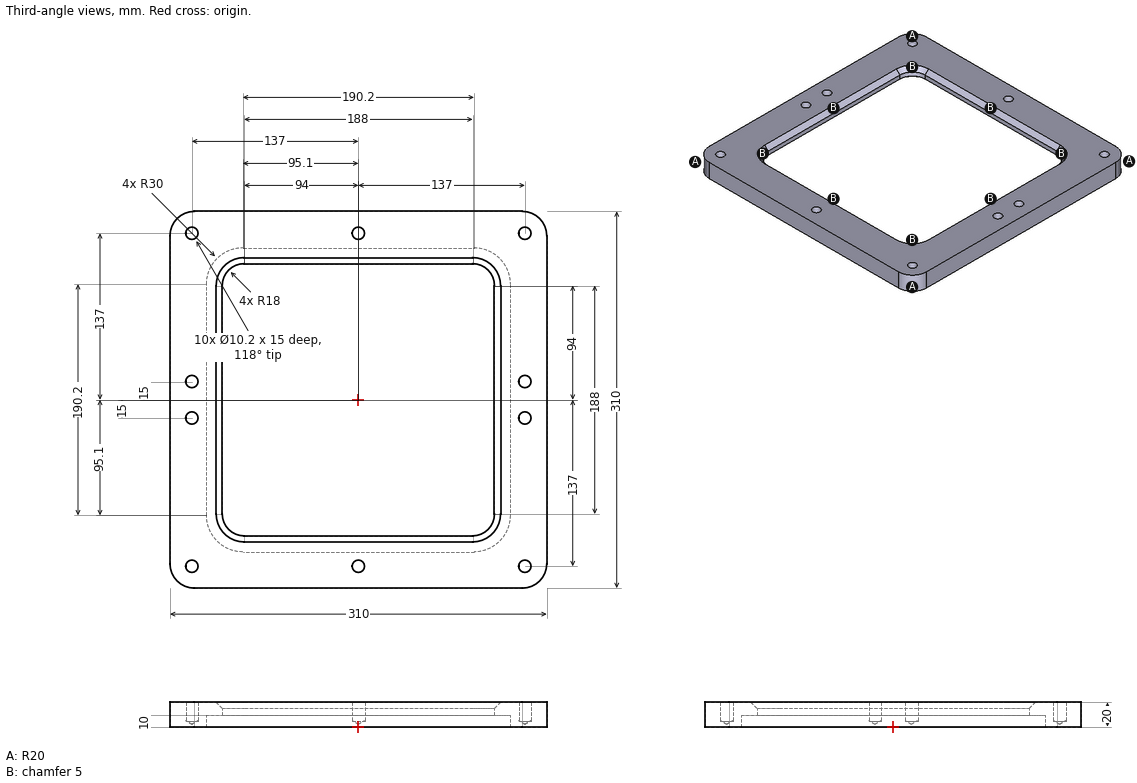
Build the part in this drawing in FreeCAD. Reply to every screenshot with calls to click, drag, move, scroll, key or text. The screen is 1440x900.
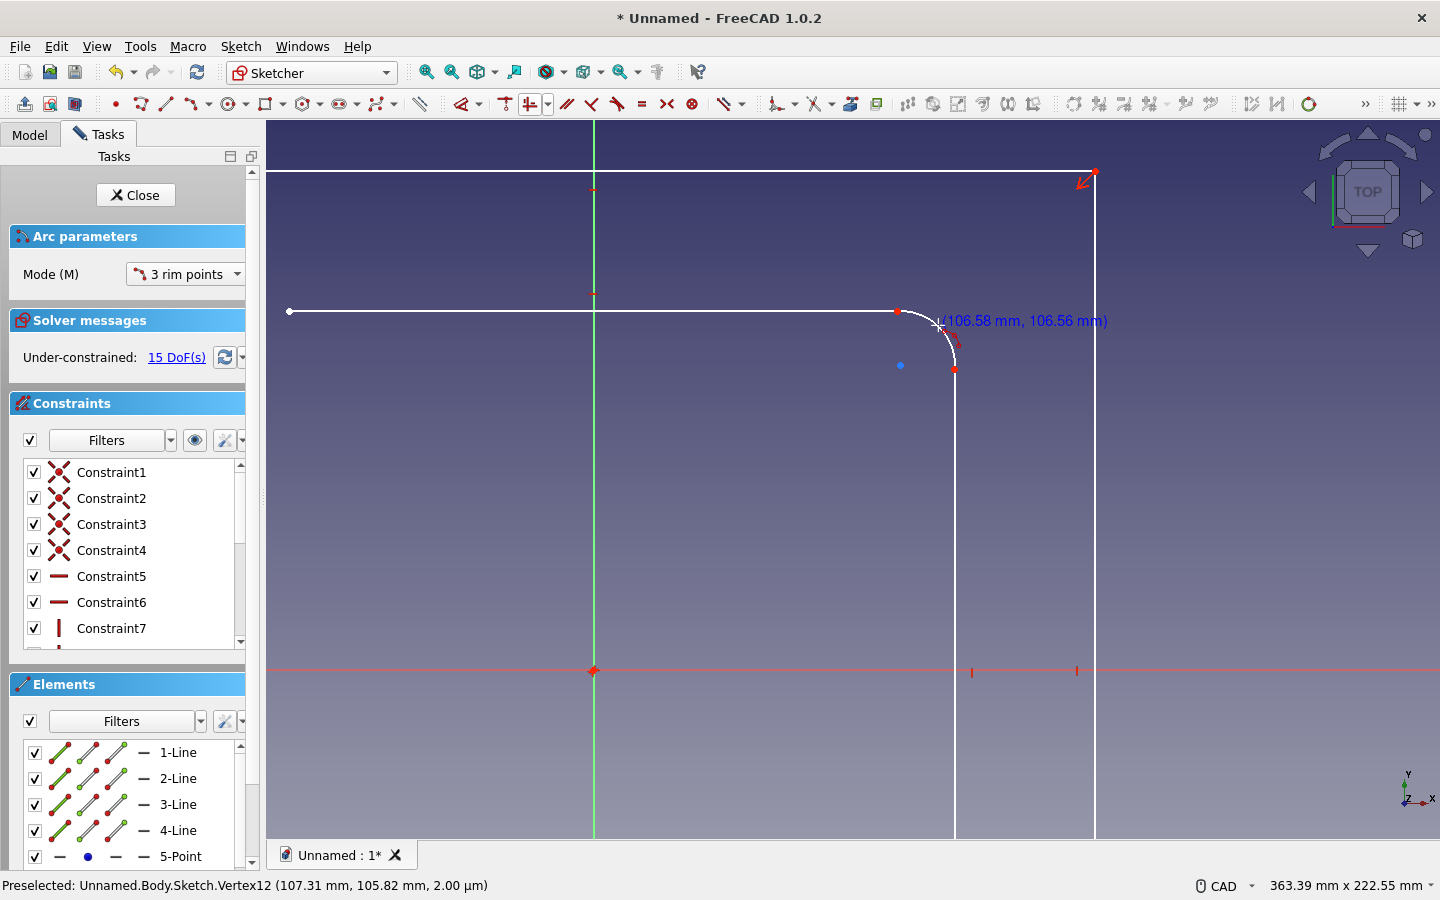
scroll(940, 324, down, 4)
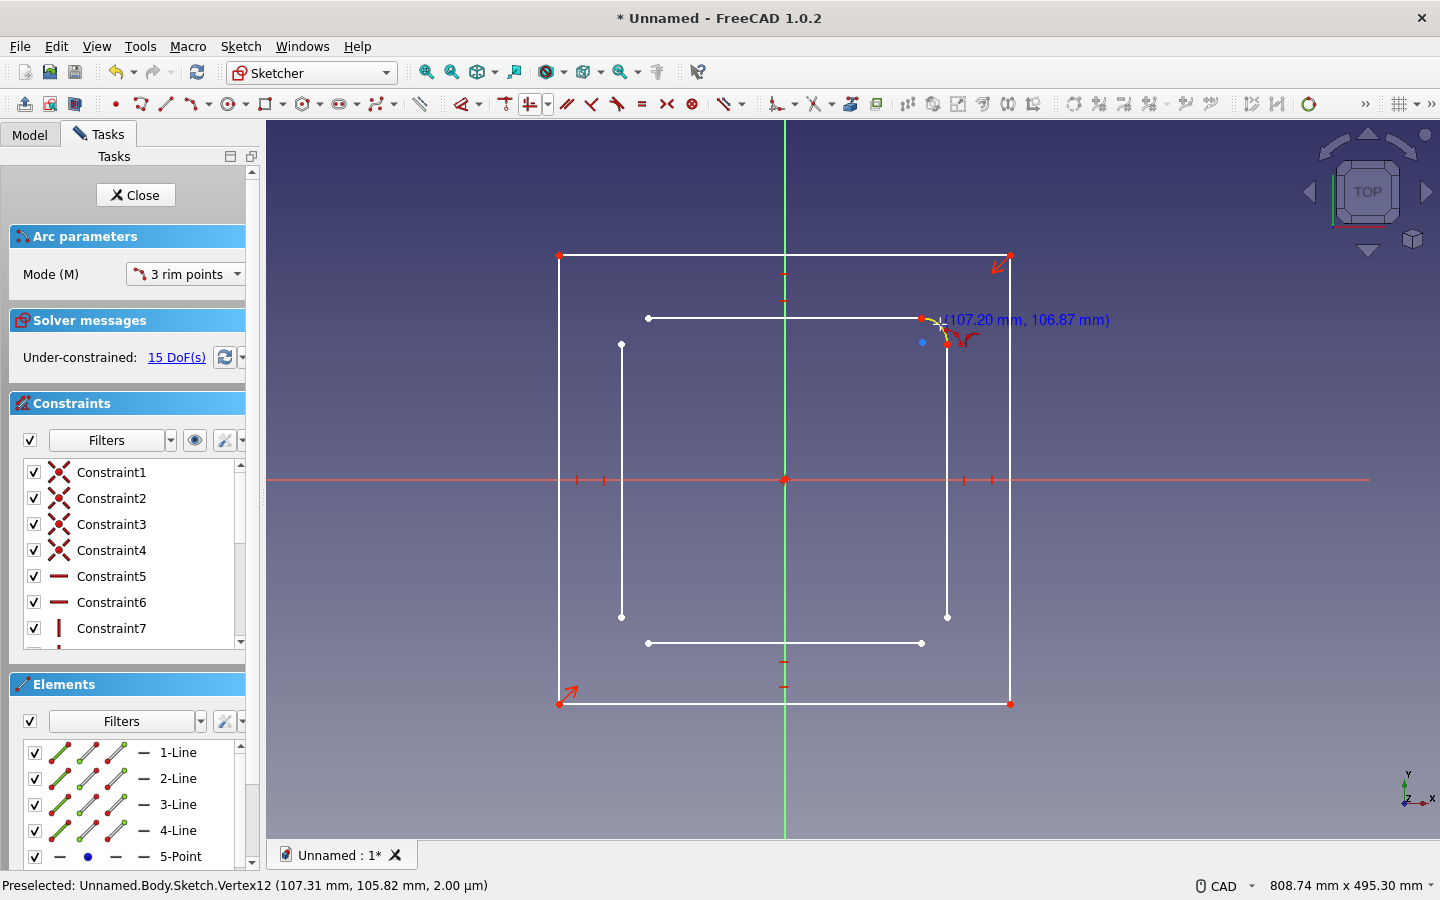
click(947, 617)
click(921, 643)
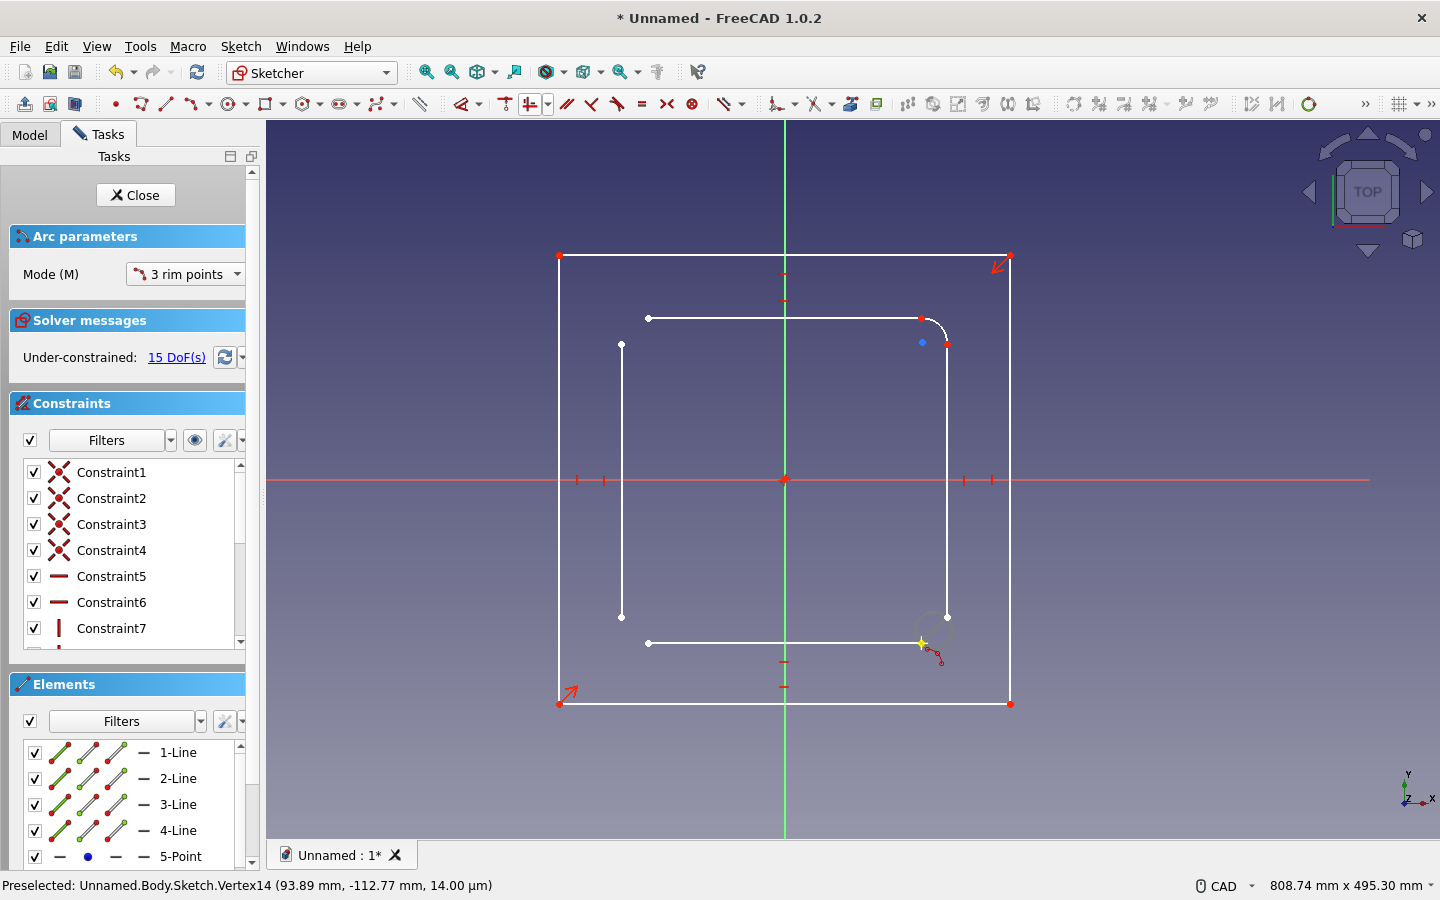
scroll(940, 635, up, 4)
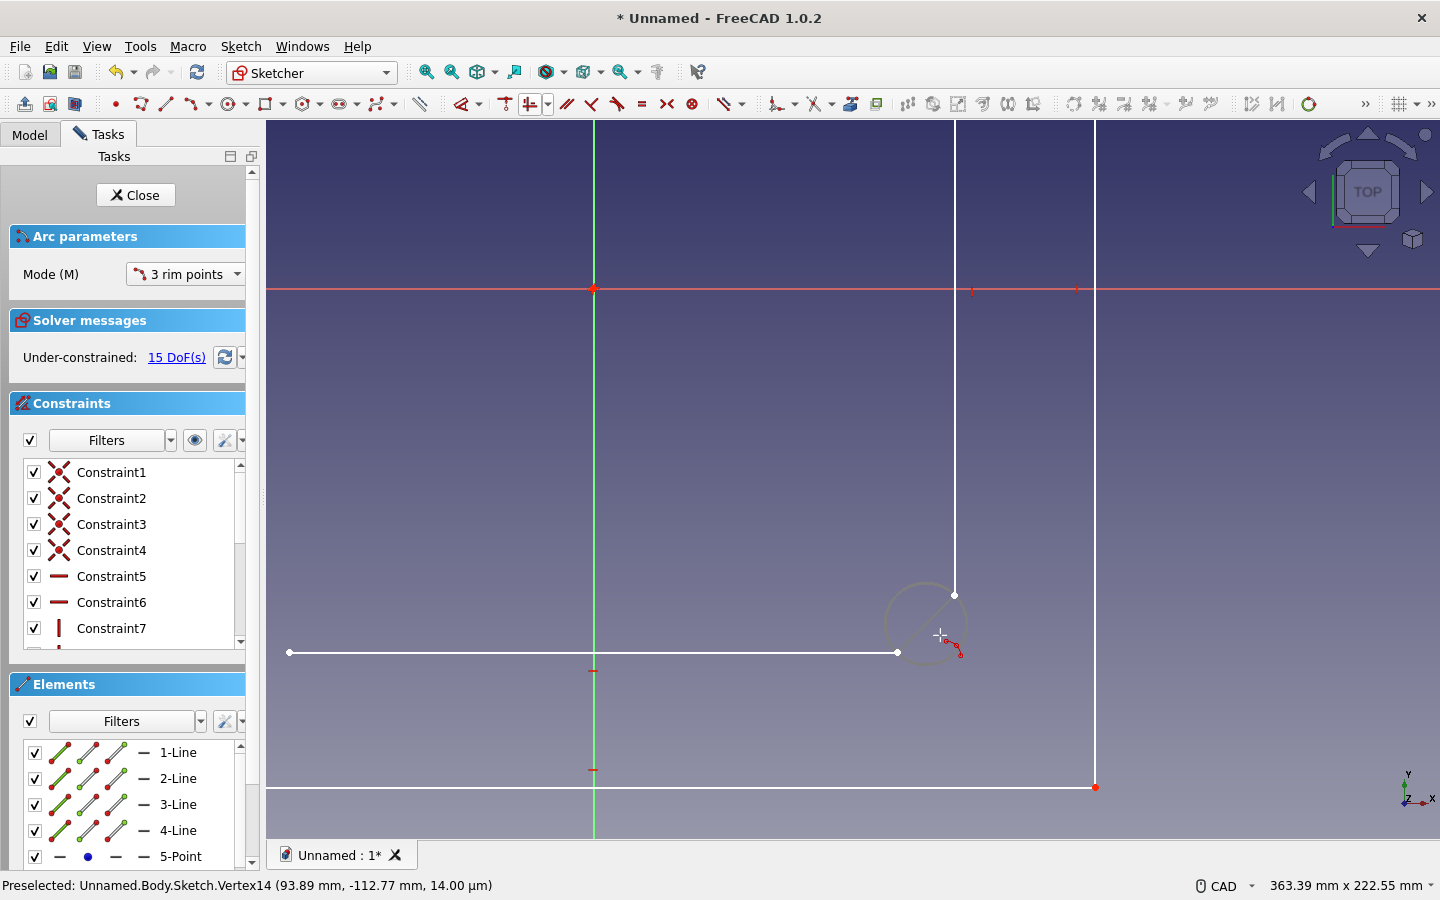
click(938, 633)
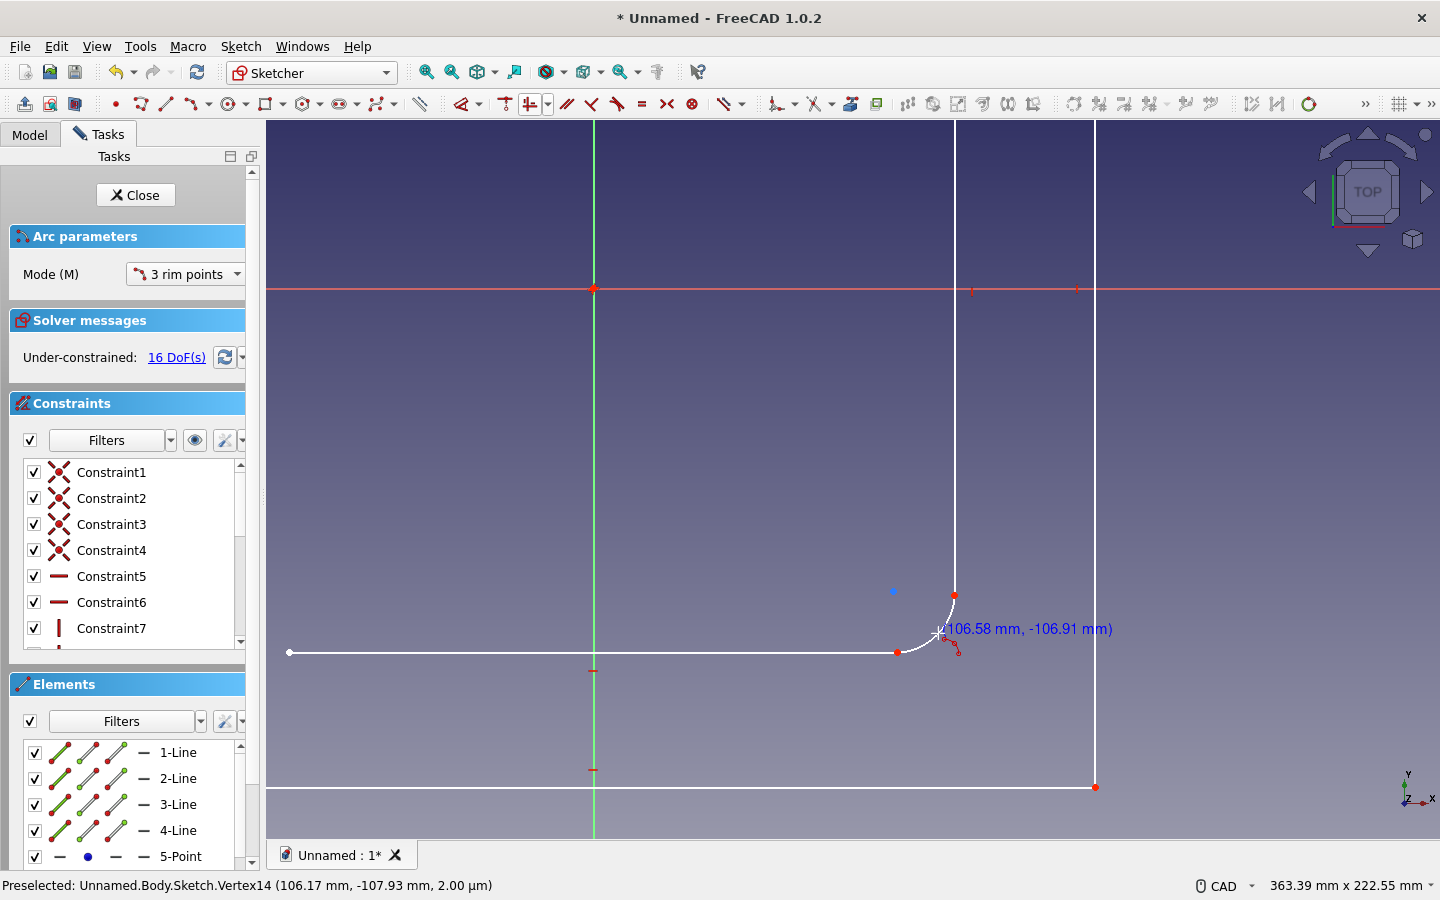
scroll(940, 635, down, 4)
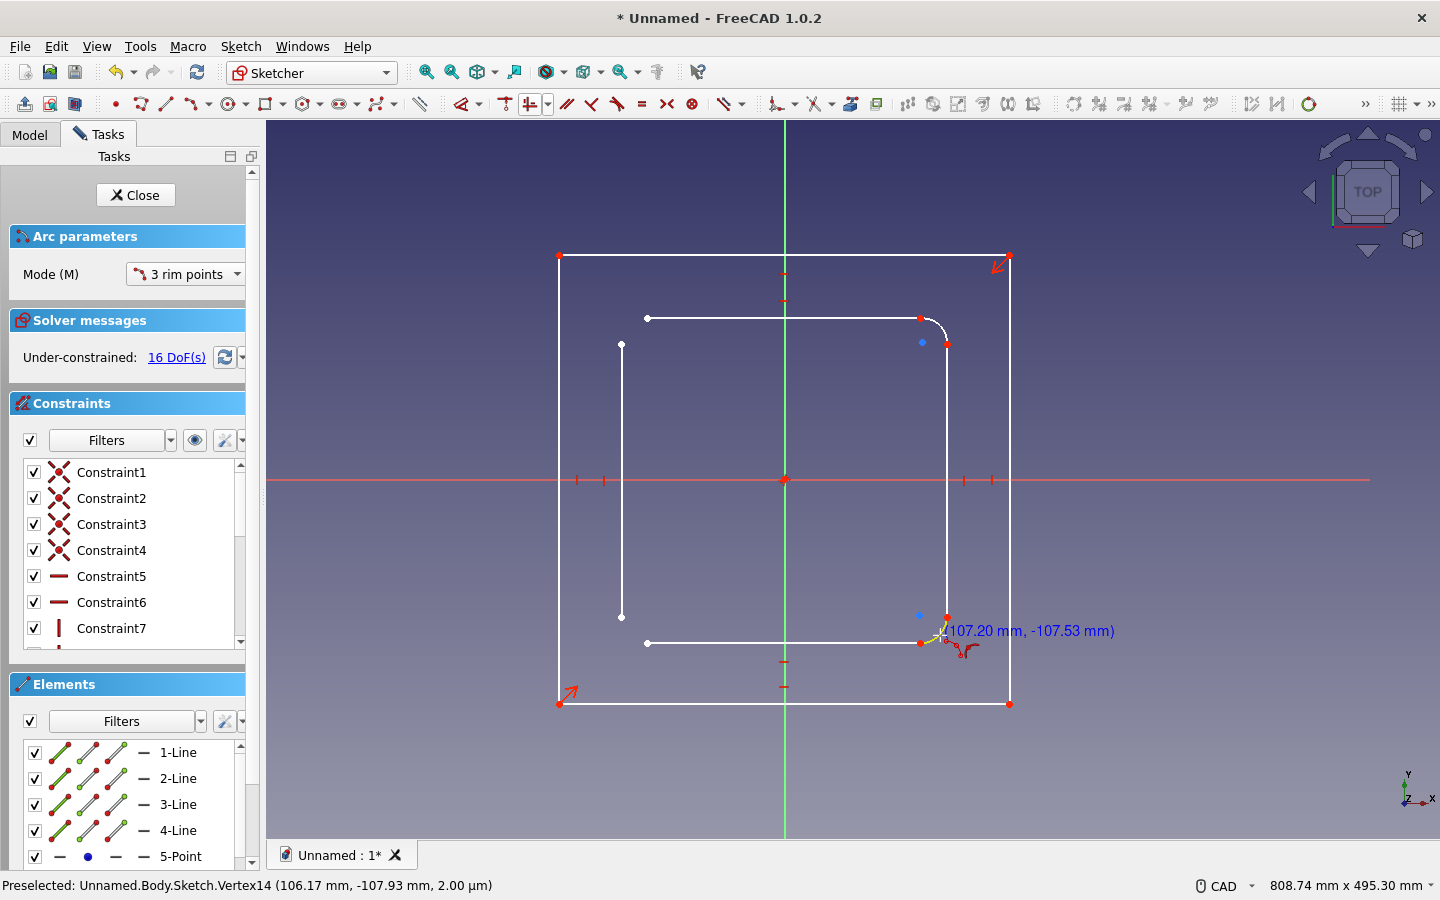
click(648, 643)
click(622, 617)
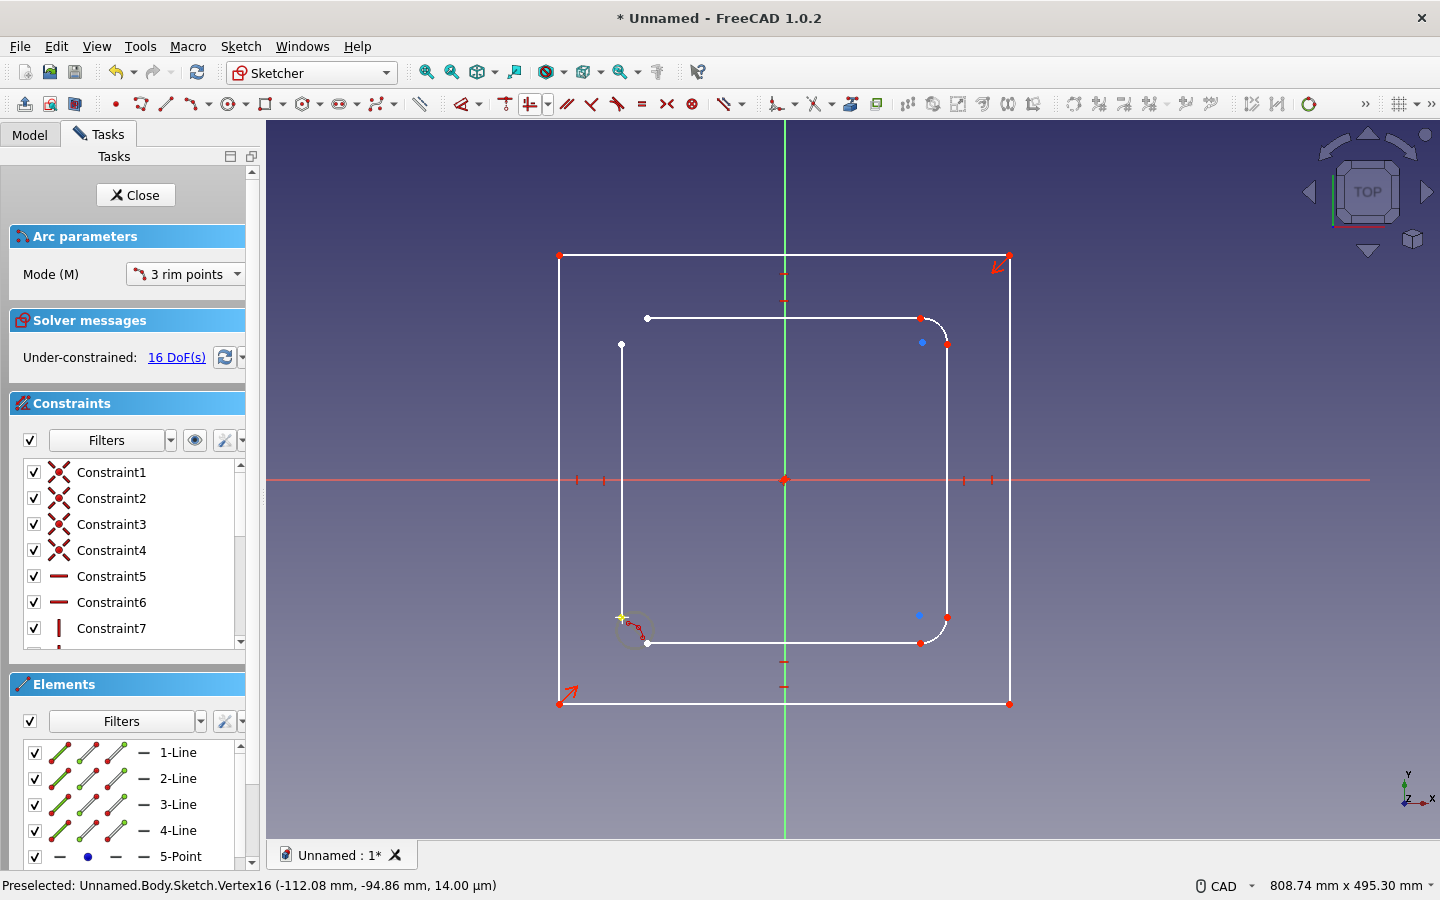
scroll(630, 635, up, 4)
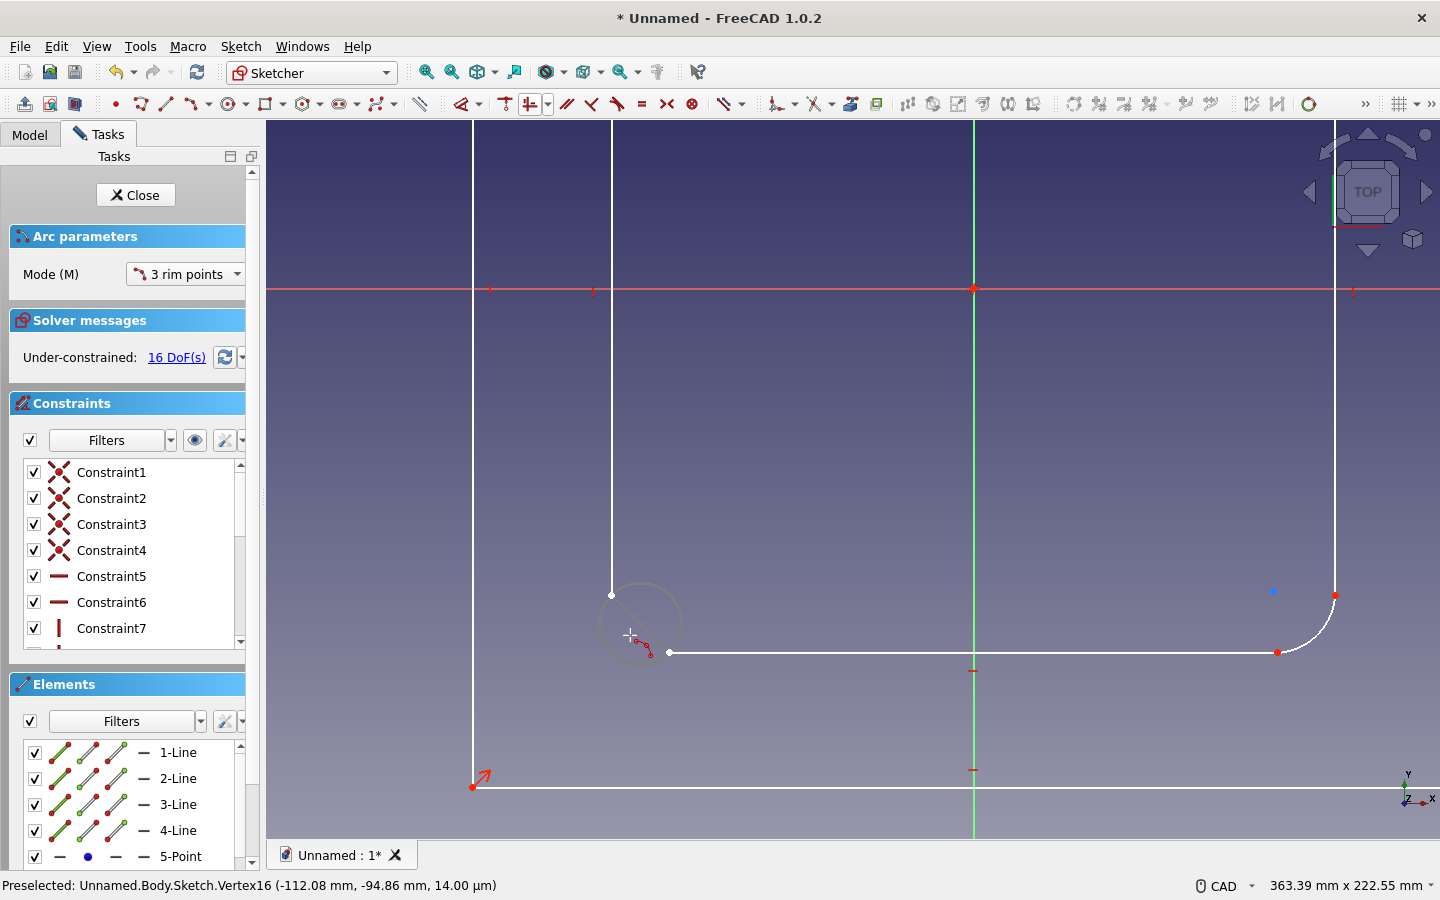
click(629, 633)